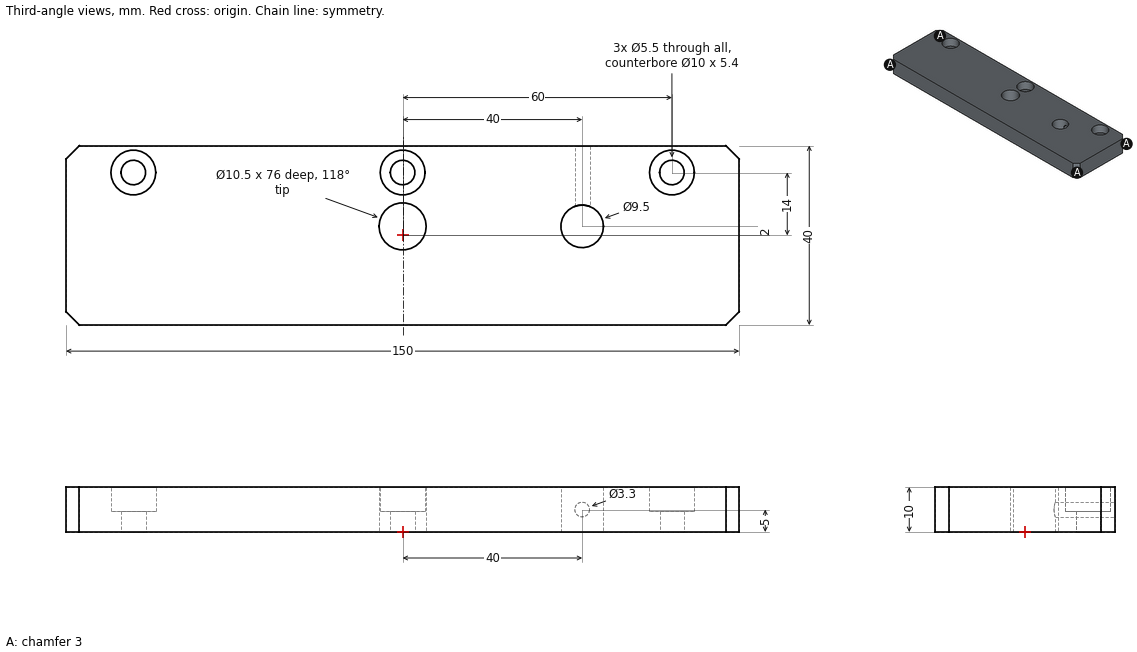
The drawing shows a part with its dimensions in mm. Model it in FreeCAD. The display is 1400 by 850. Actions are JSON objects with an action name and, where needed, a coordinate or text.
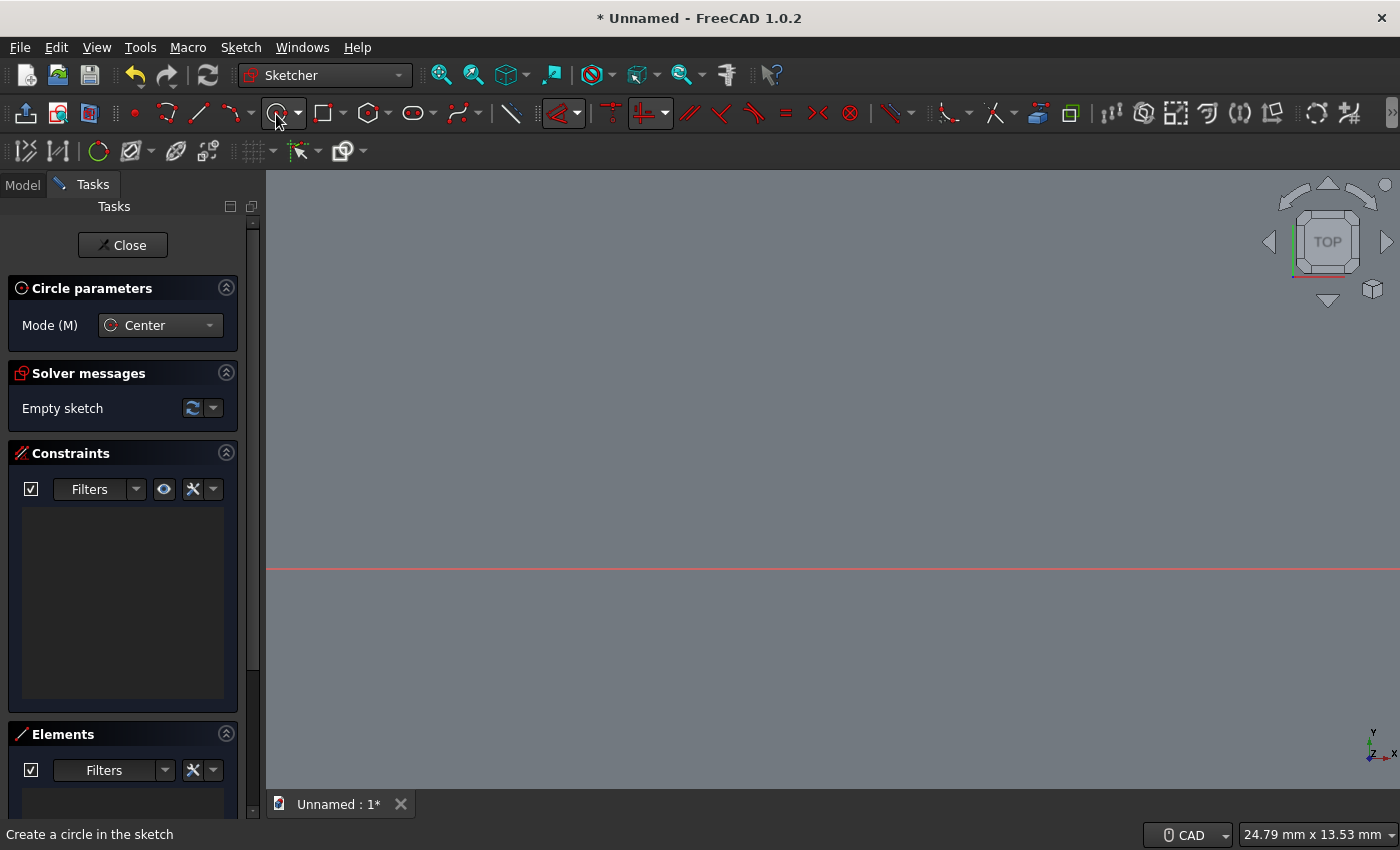
{"action": "left_click", "coordinate": [760, 478]}
{"action": "mouse_move", "coordinate": [914, 324]}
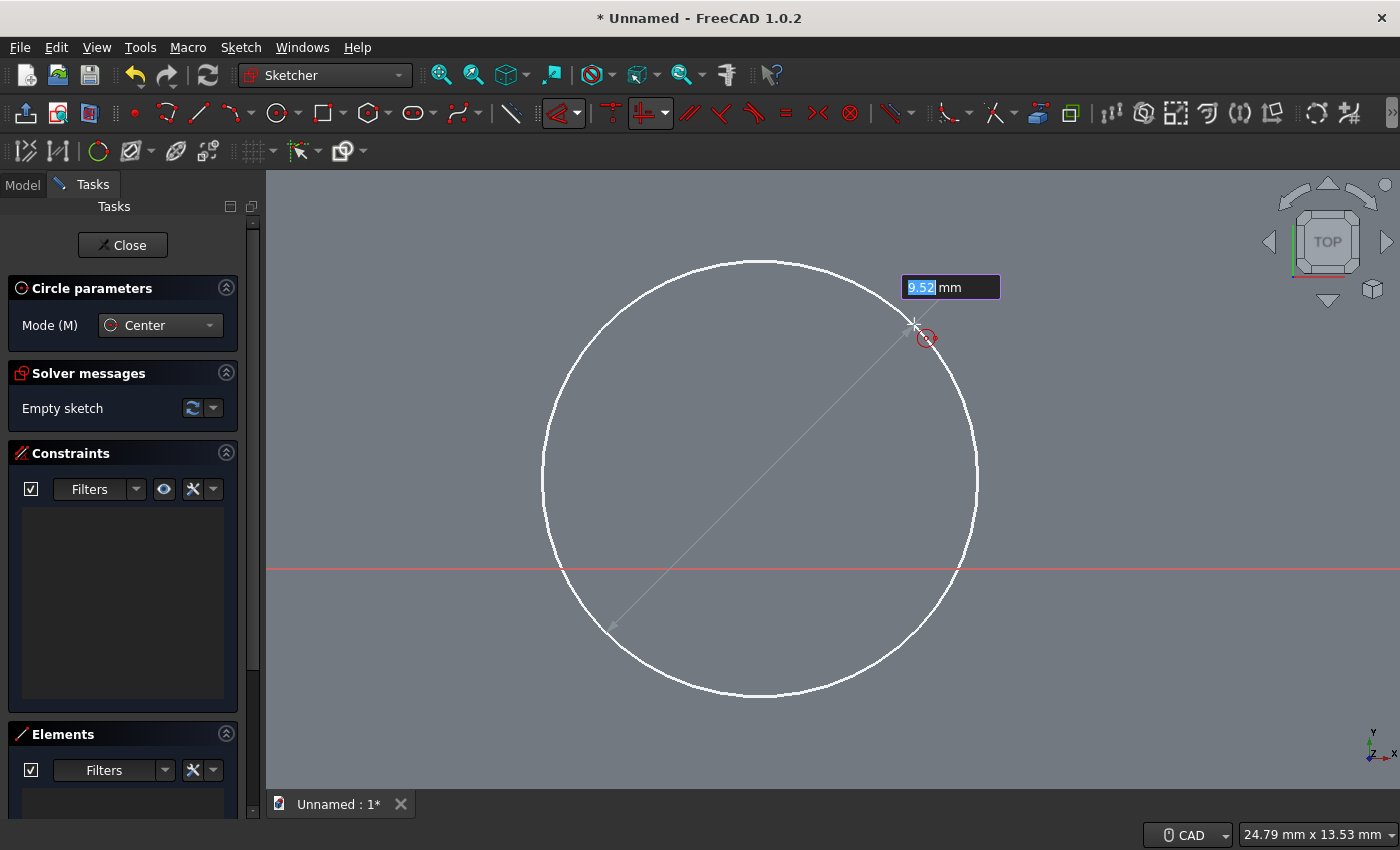
{"action": "type", "text": "9.5"}
{"action": "key", "text": "Return"}
{"action": "key", "text": "Escape"}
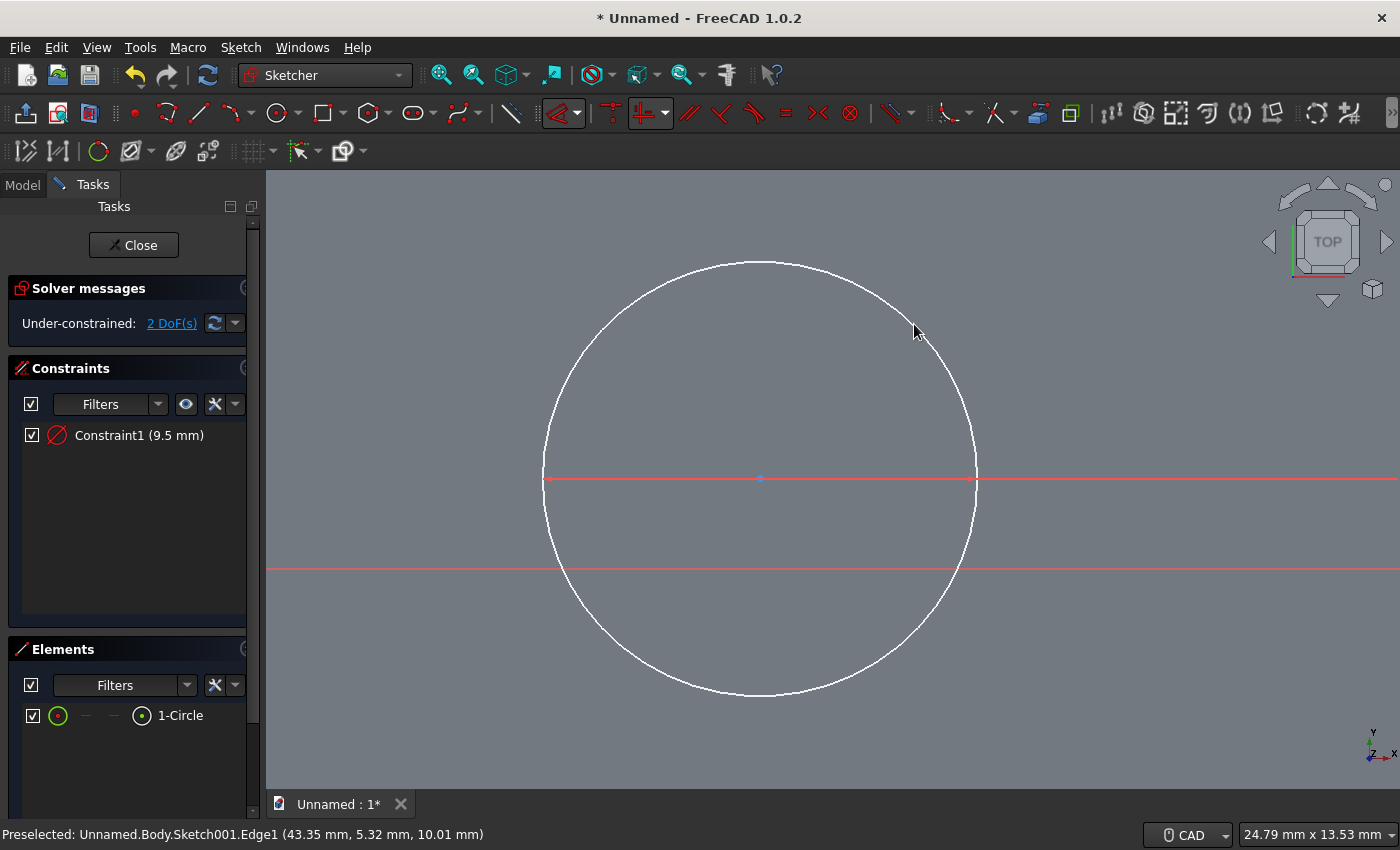
{"action": "key", "text": "d"}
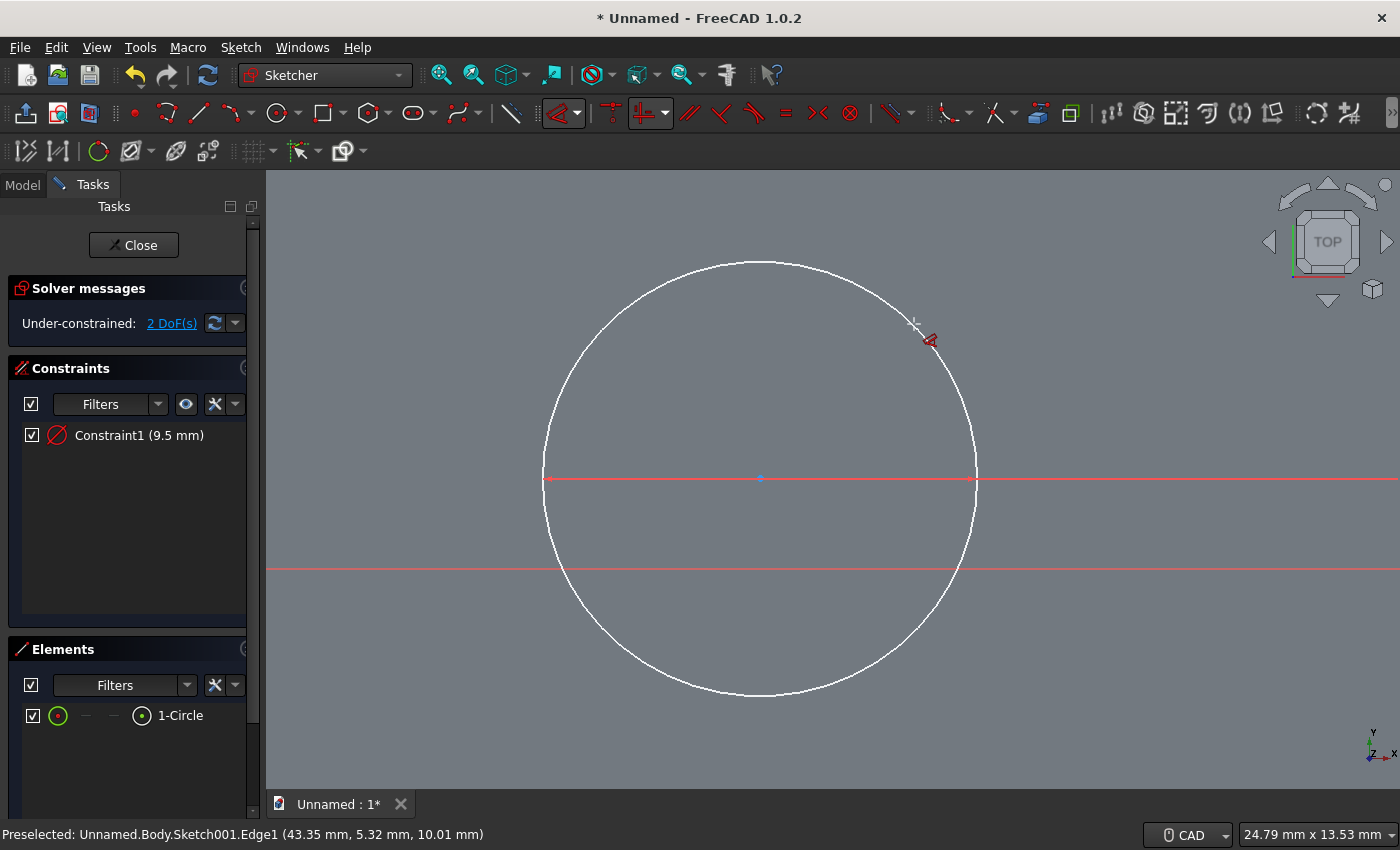
{"action": "left_click", "coordinate": [760, 479]}
{"action": "left_click", "coordinate": [794, 524]}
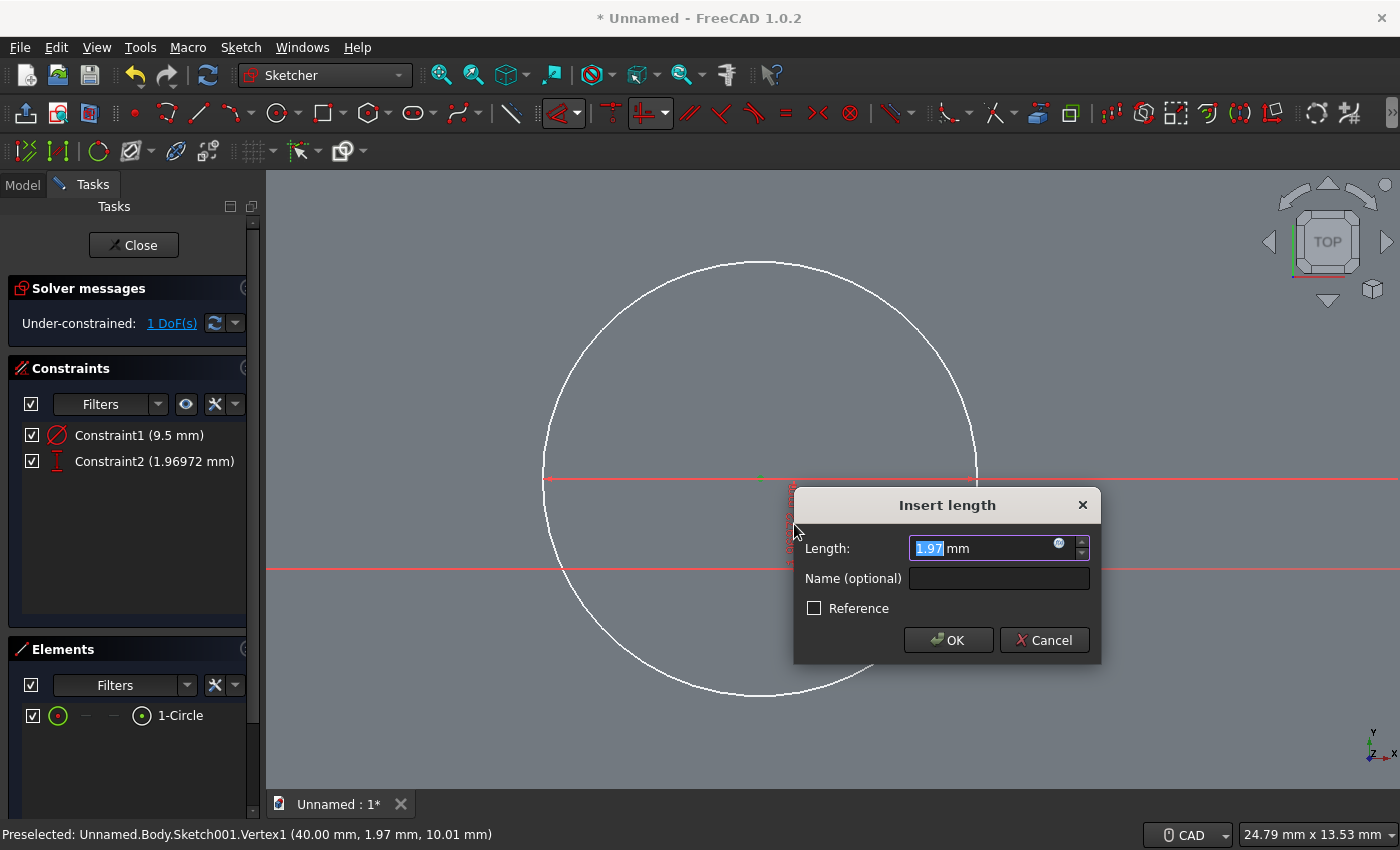
{"action": "type", "text": "2"}
{"action": "key", "text": "Return"}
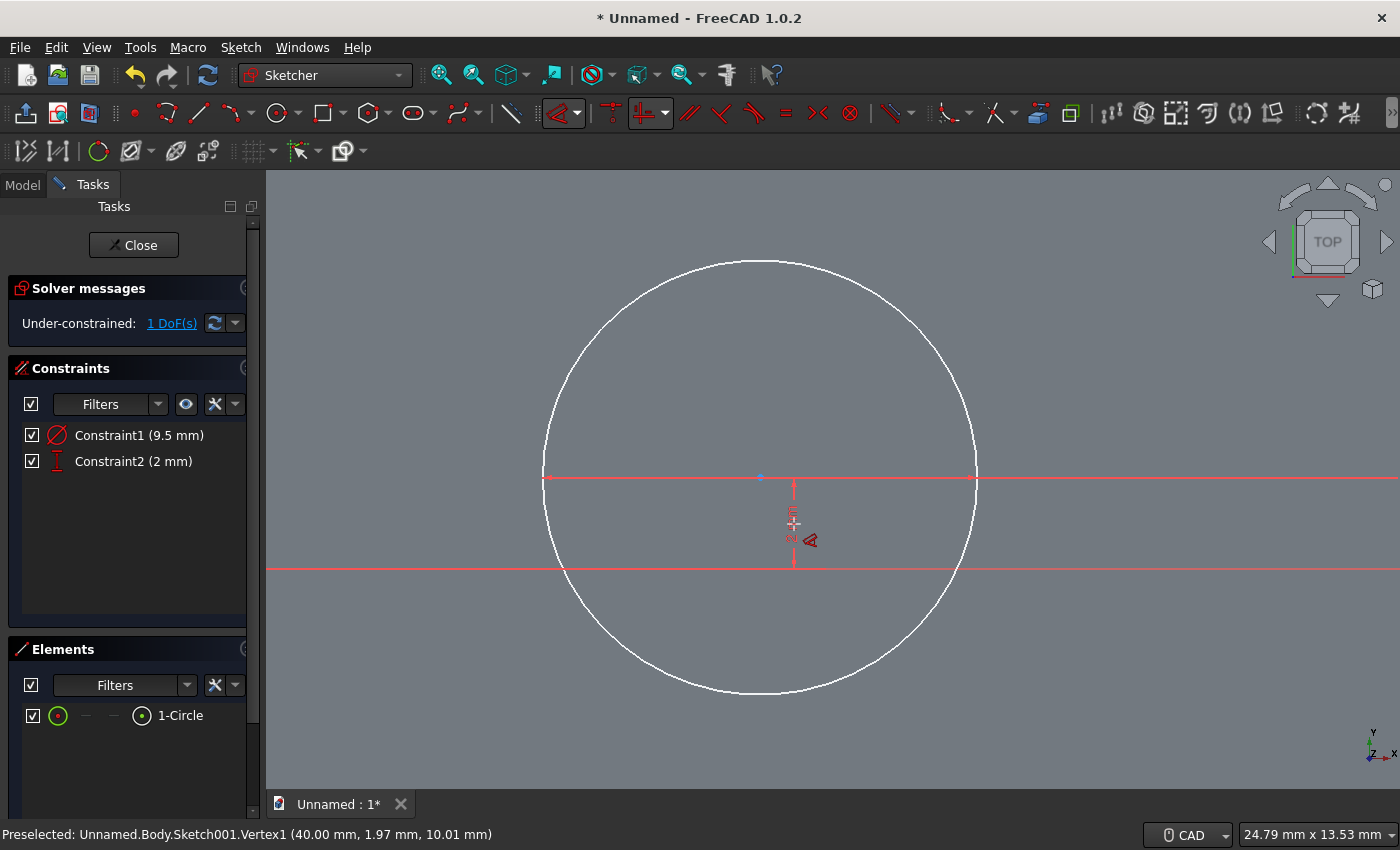
{"action": "left_click", "coordinate": [760, 478]}
{"action": "left_click", "coordinate": [527, 603]}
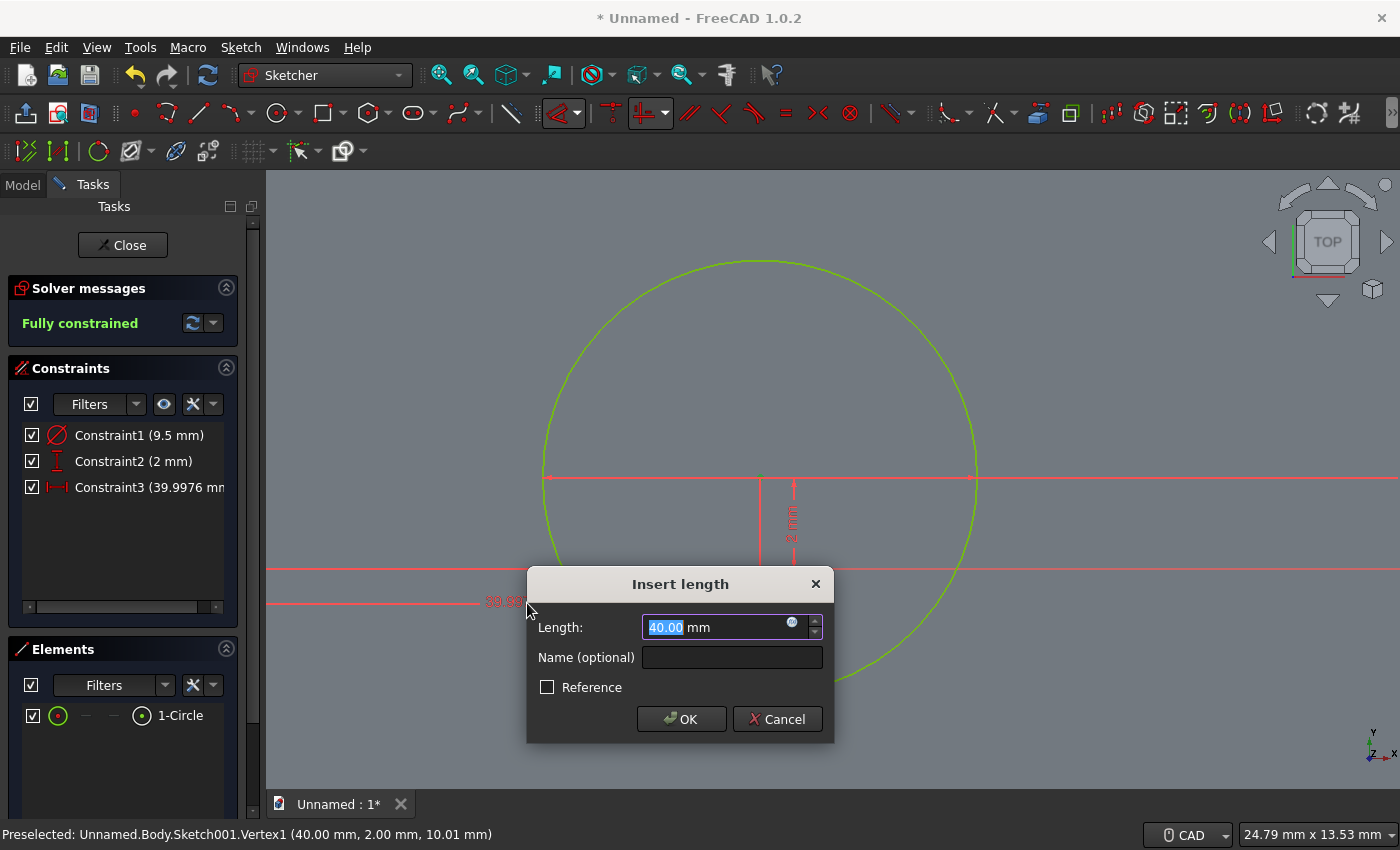
{"action": "type", "text": "40"}
{"action": "key", "text": "Return"}
{"action": "key", "text": "Escape"}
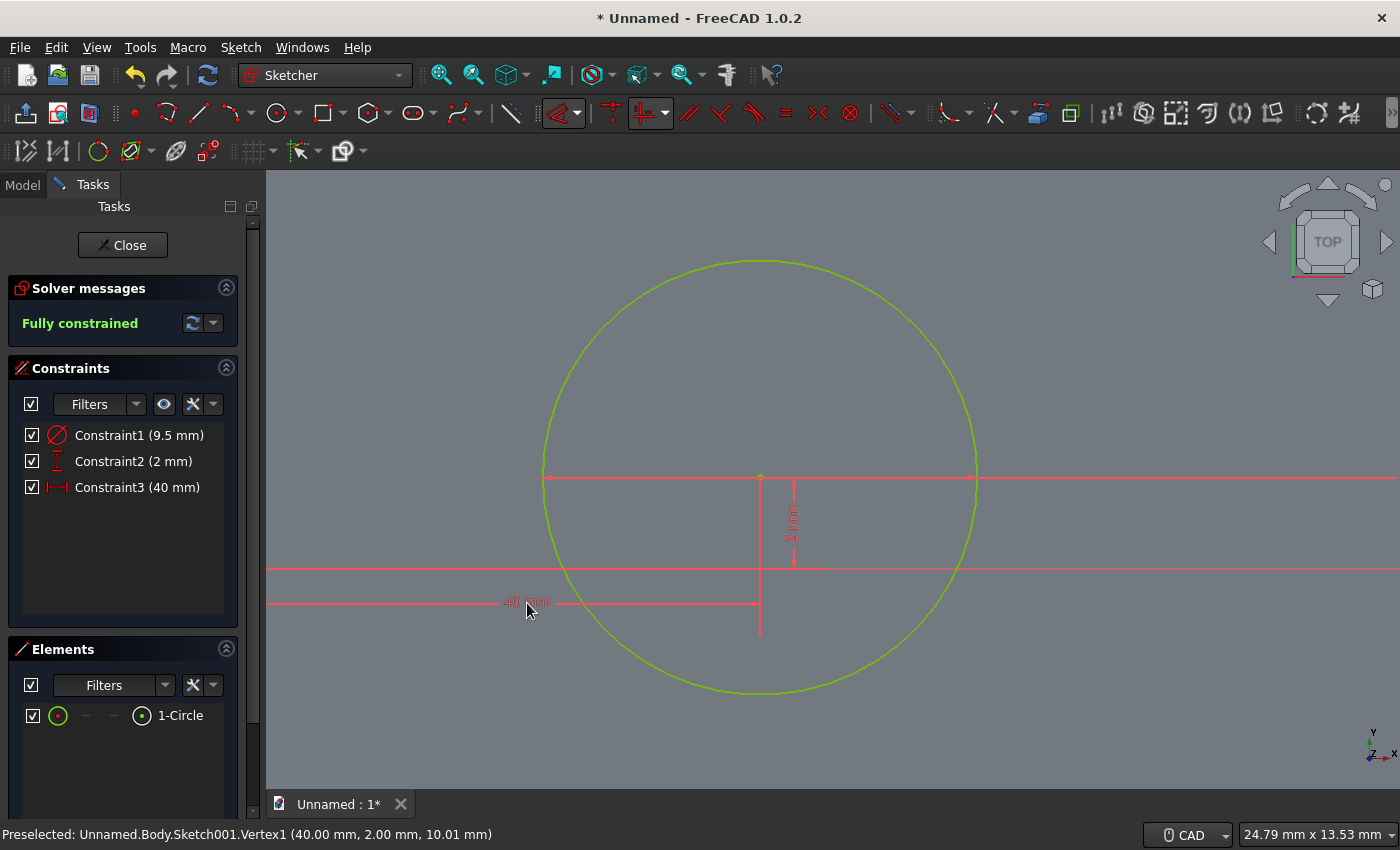
{"action": "left_click", "coordinate": [123, 245]}